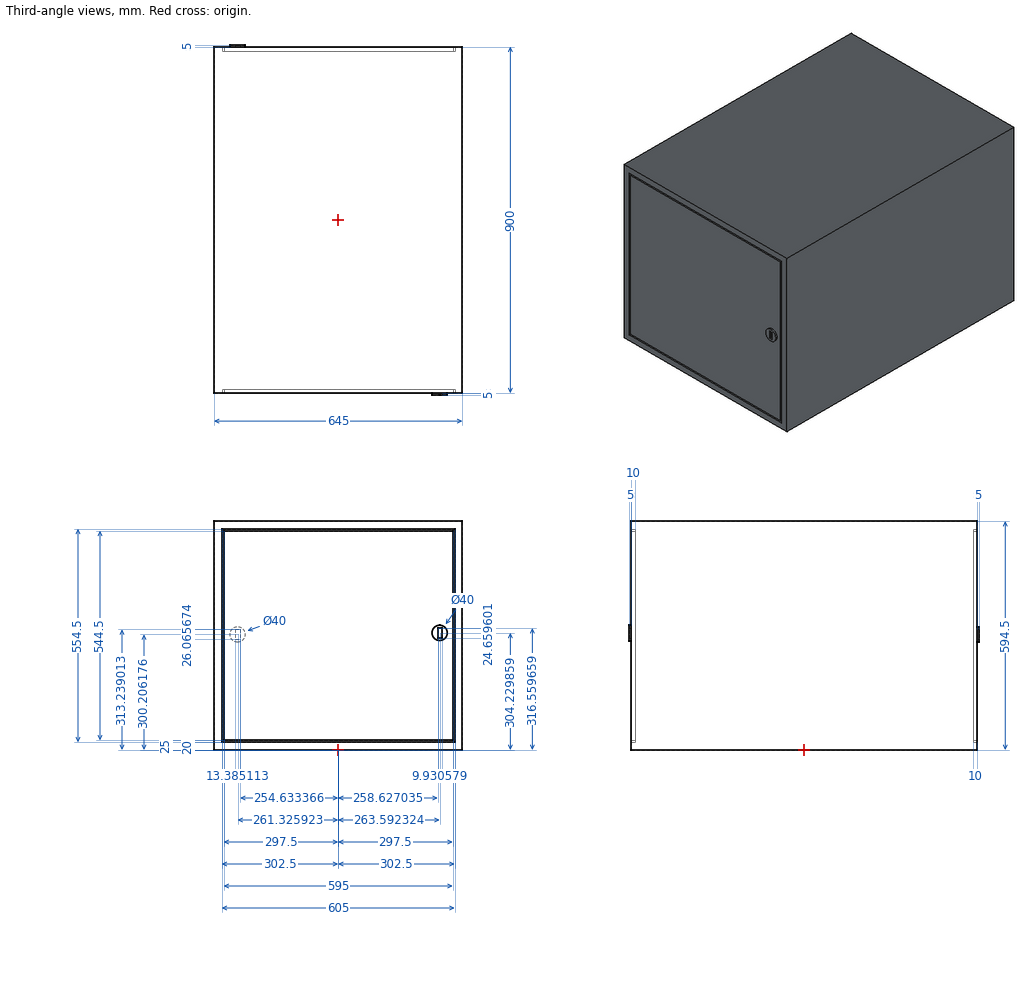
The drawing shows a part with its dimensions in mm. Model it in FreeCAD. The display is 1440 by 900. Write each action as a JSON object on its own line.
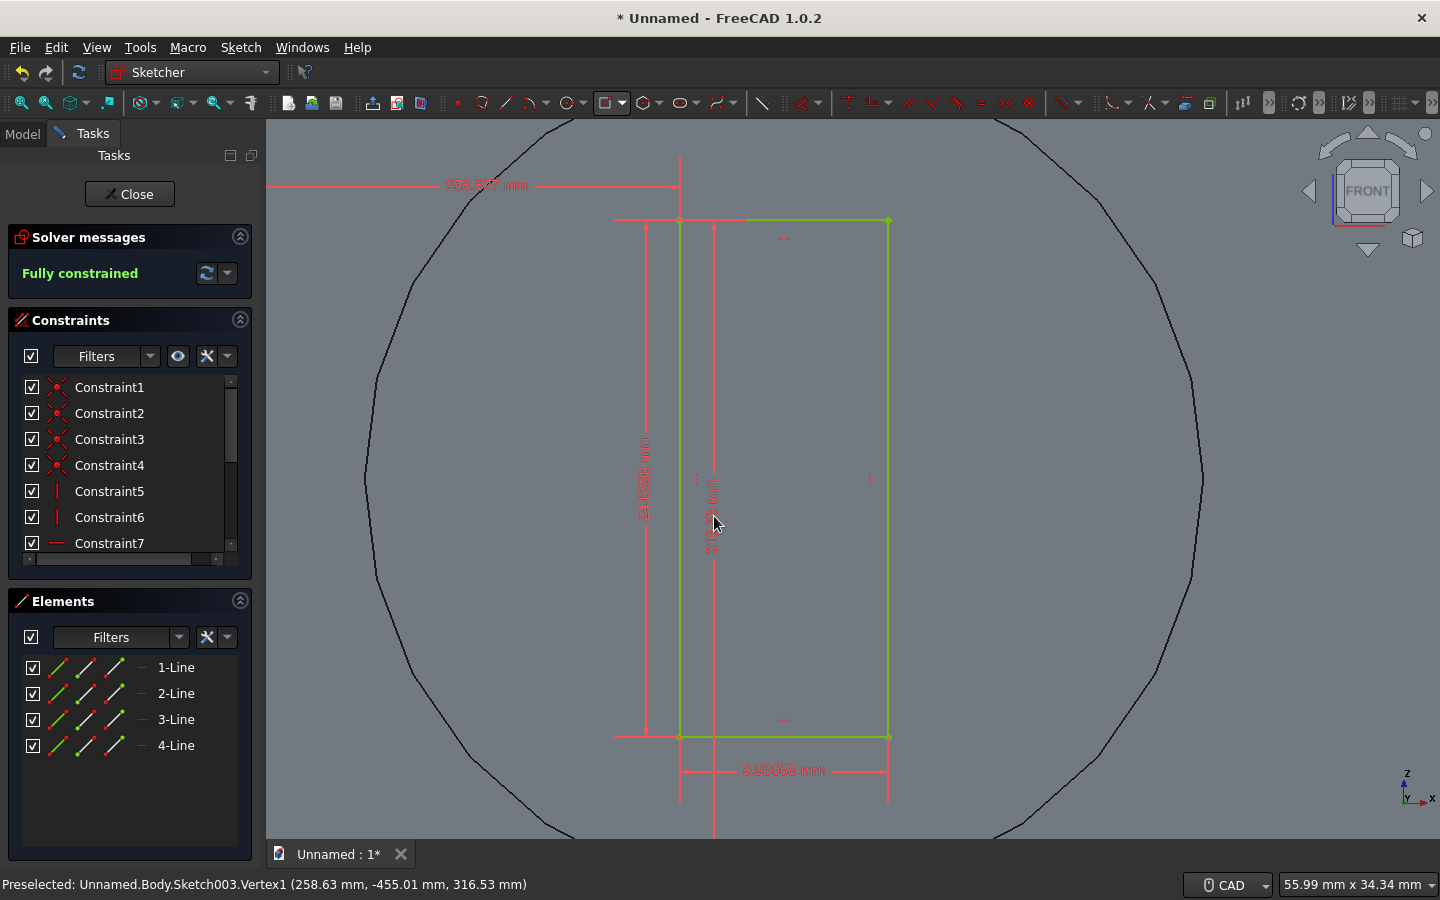
{"action": "left_click", "coordinate": [130, 194]}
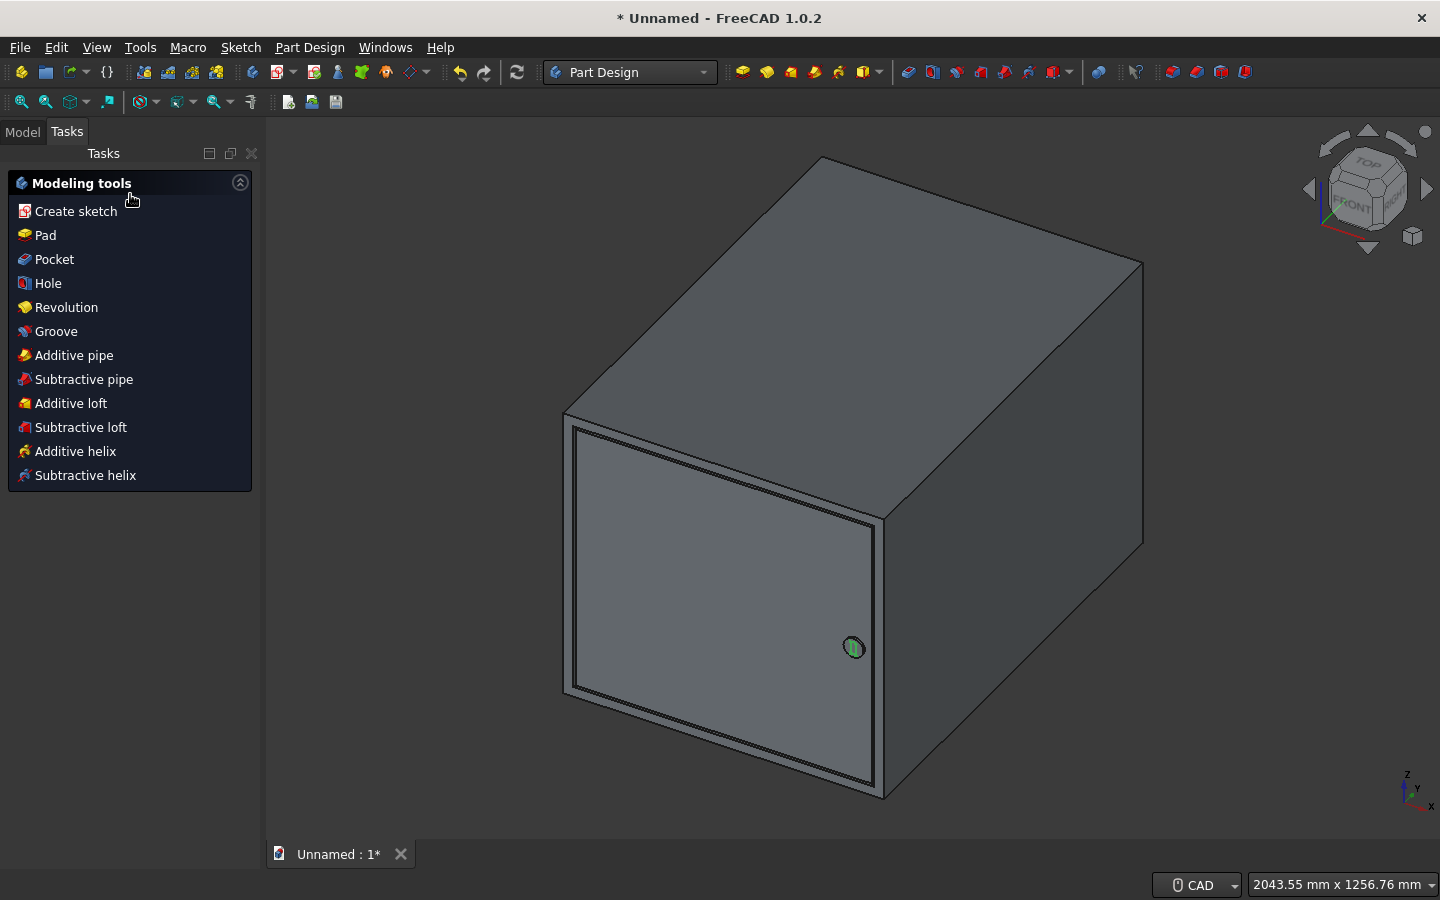
{"action": "left_click", "coordinate": [910, 72]}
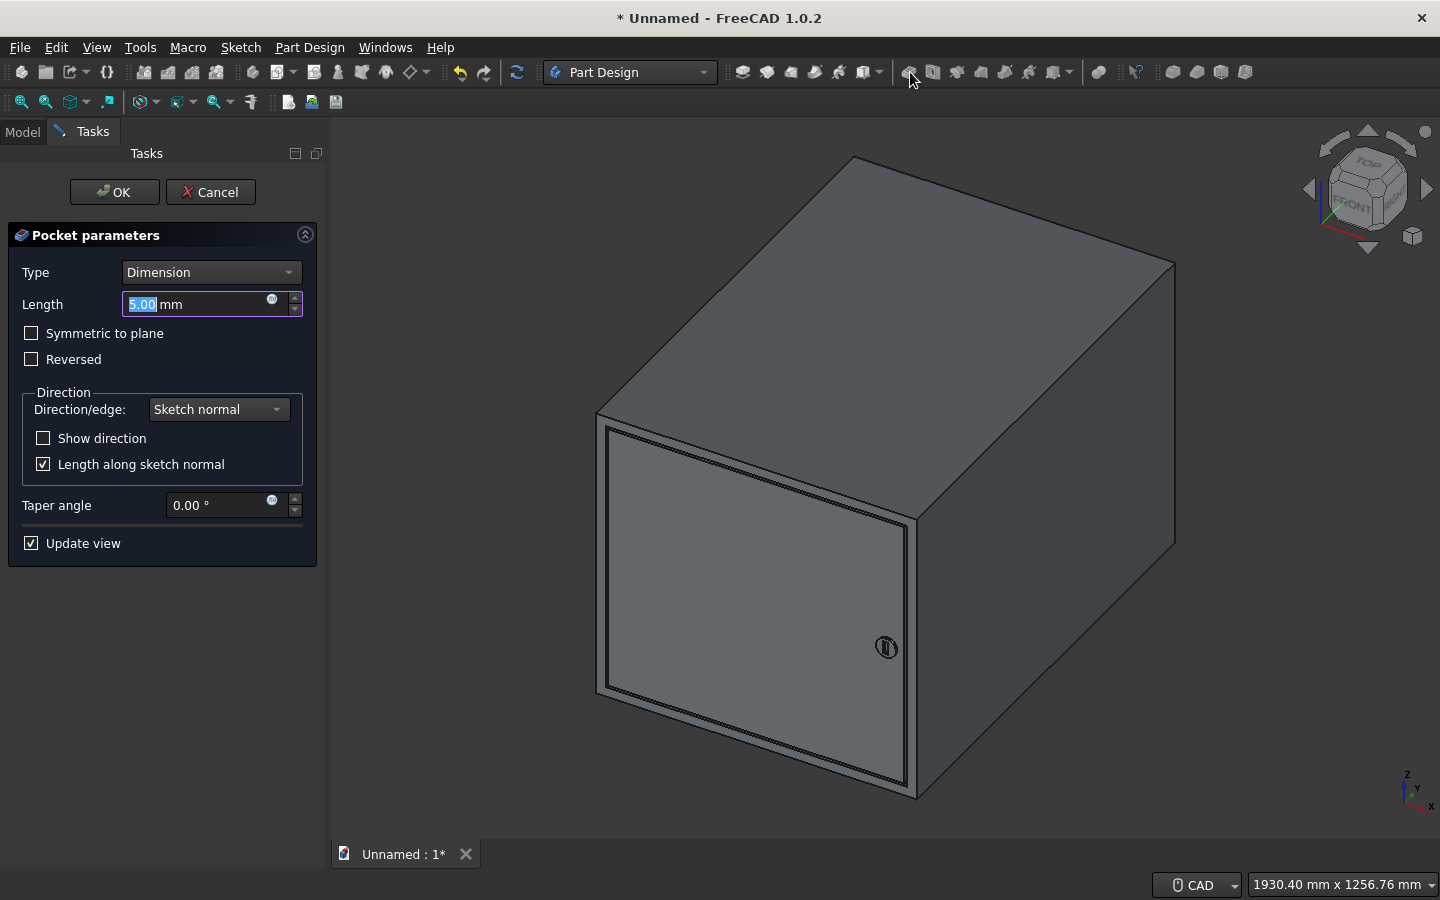
{"action": "type", "text": "5"}
{"action": "key", "text": "Tab"}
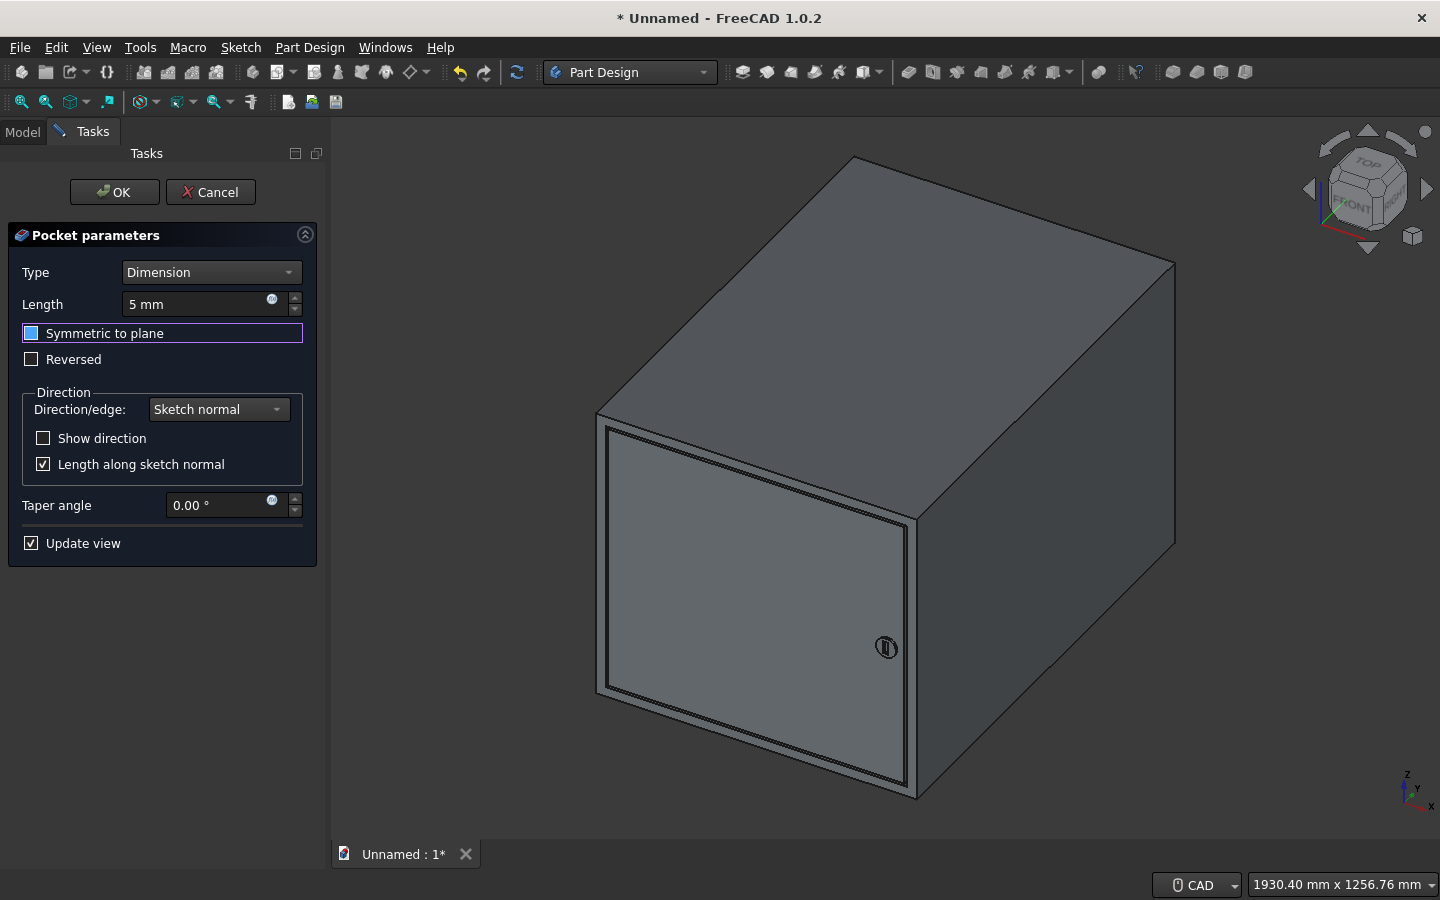
{"action": "left_click", "coordinate": [115, 192]}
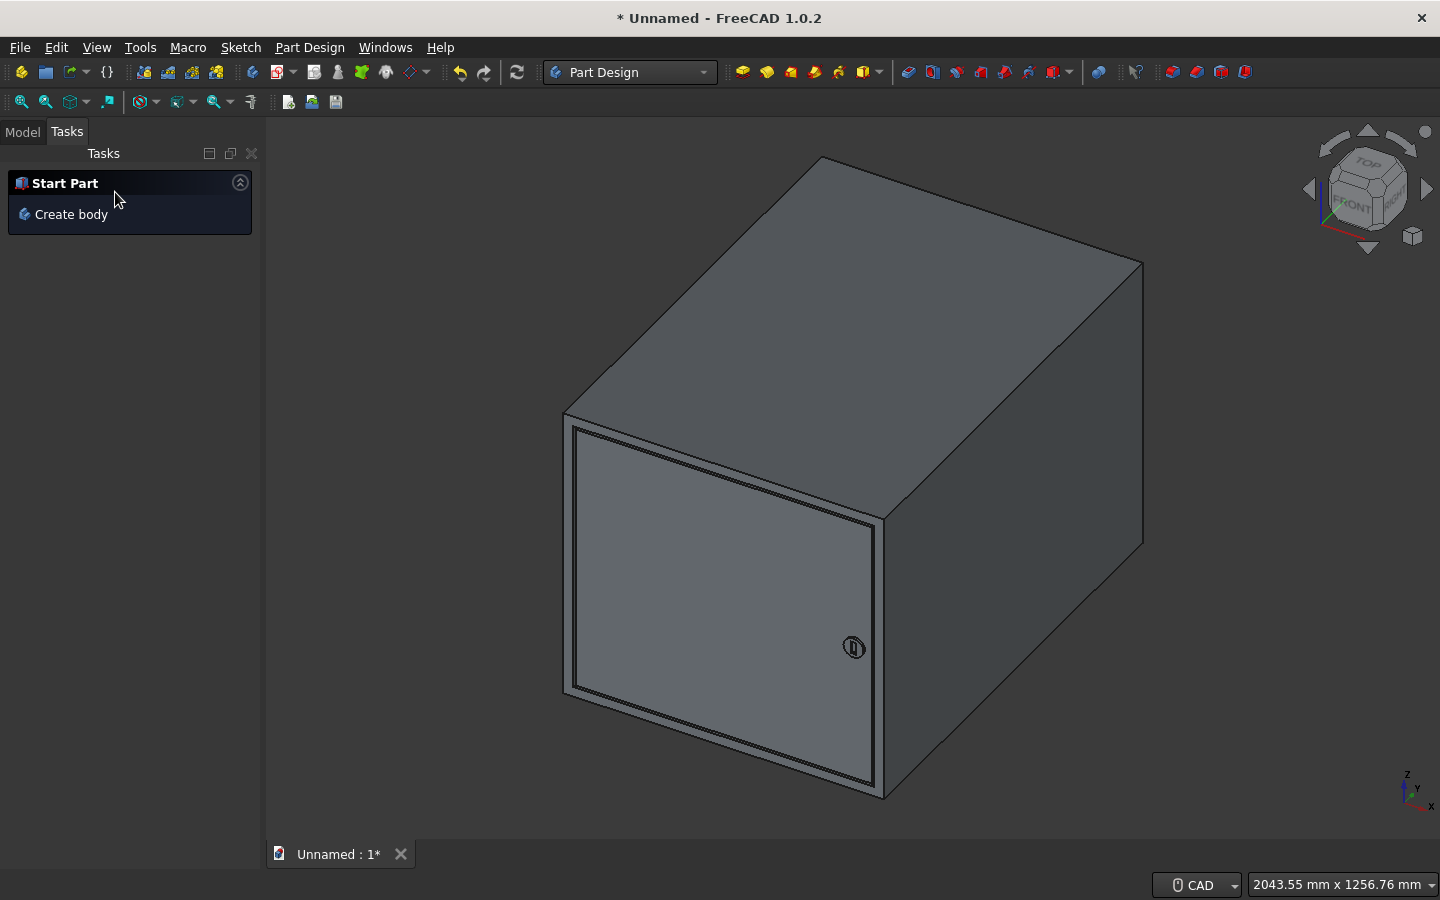
{"action": "key", "text": "4"}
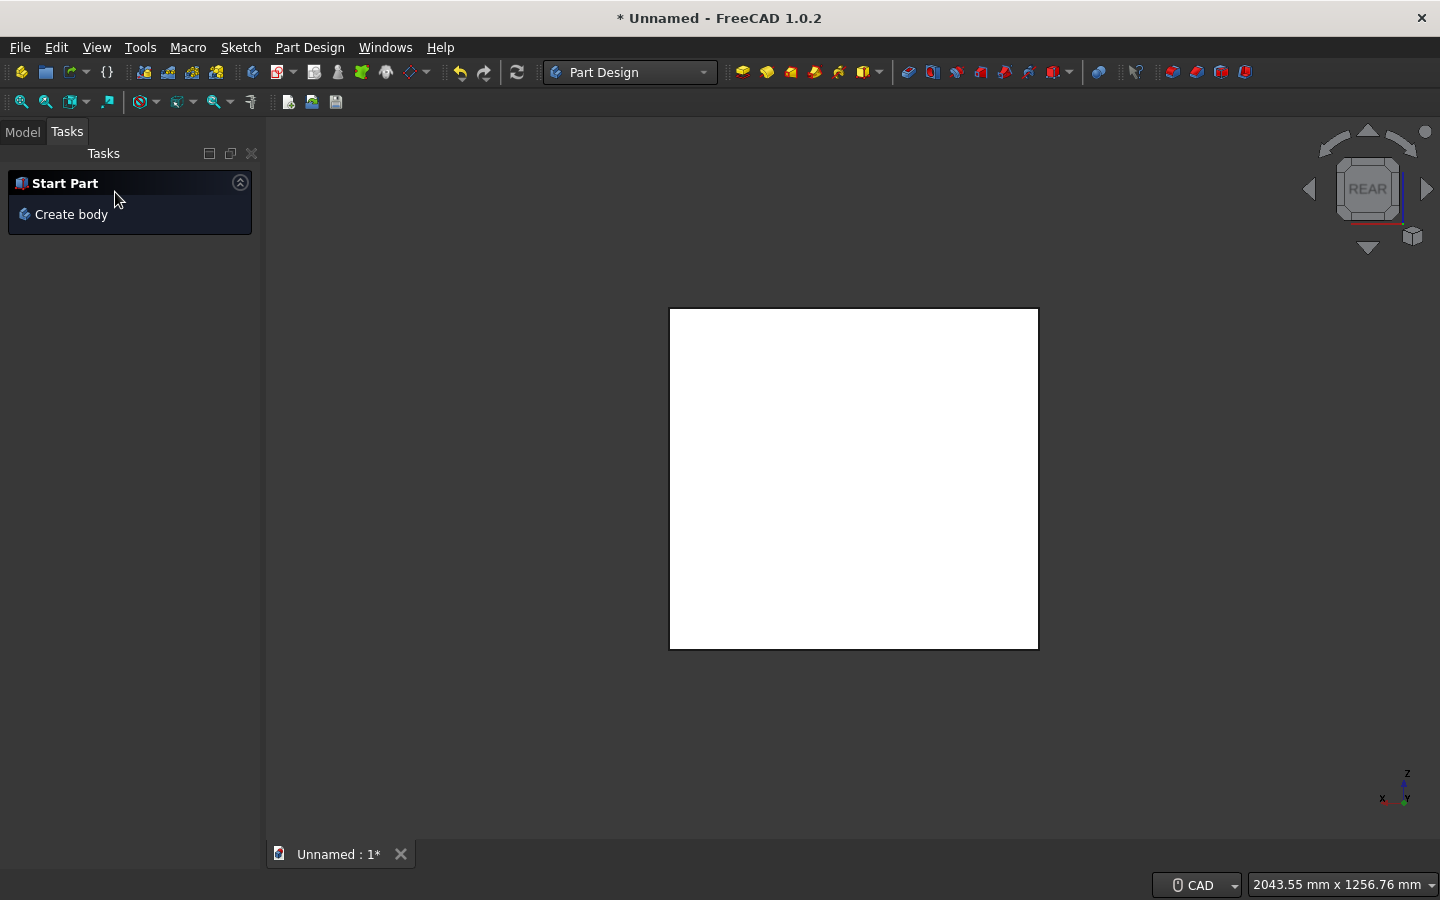
{"action": "left_click", "coordinate": [854, 478]}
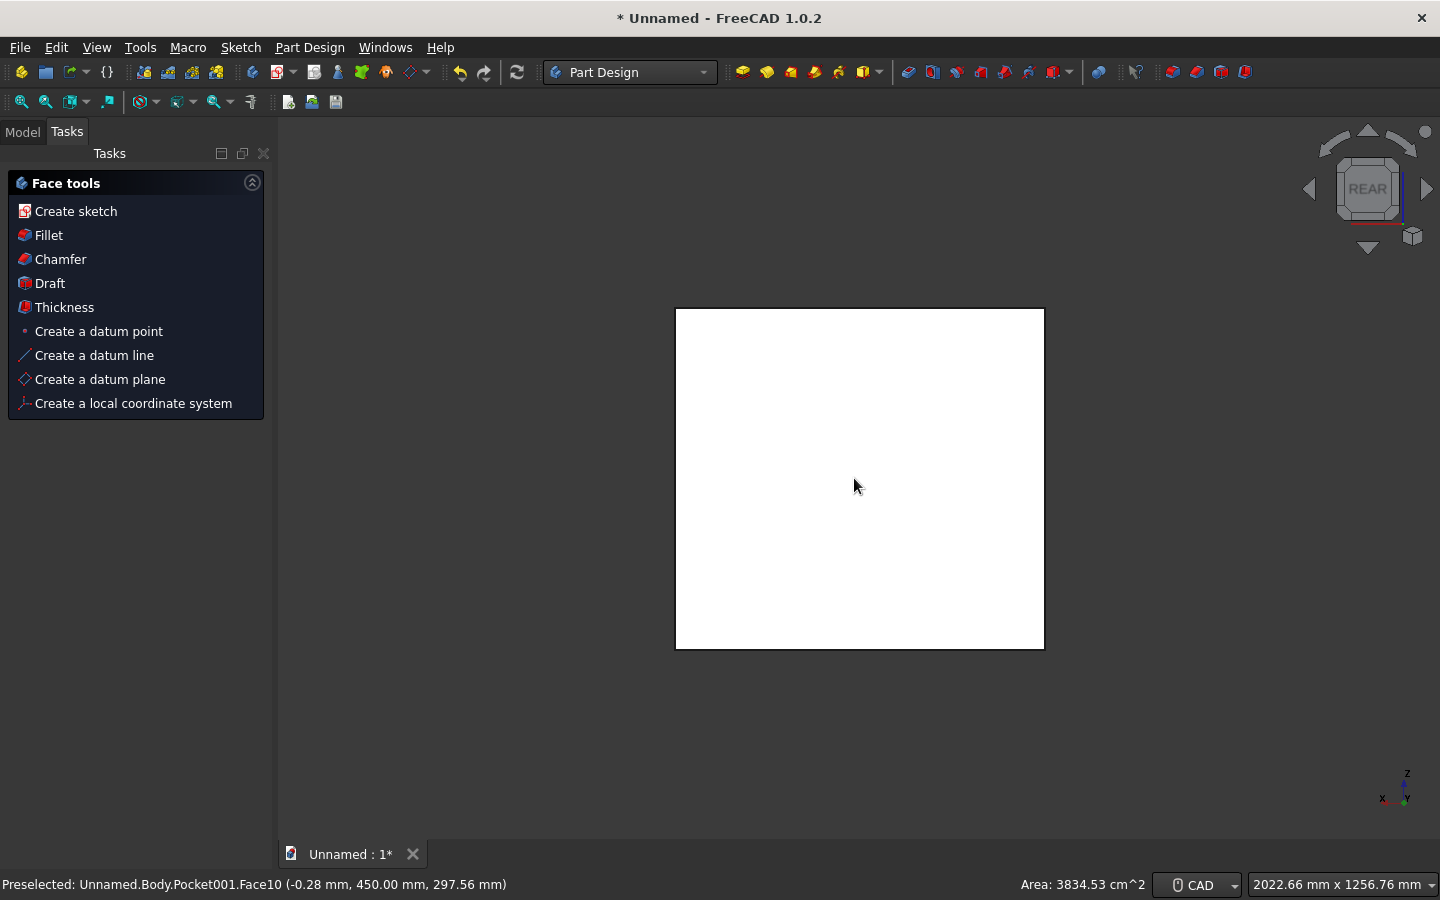
{"action": "left_click", "coordinate": [278, 72]}